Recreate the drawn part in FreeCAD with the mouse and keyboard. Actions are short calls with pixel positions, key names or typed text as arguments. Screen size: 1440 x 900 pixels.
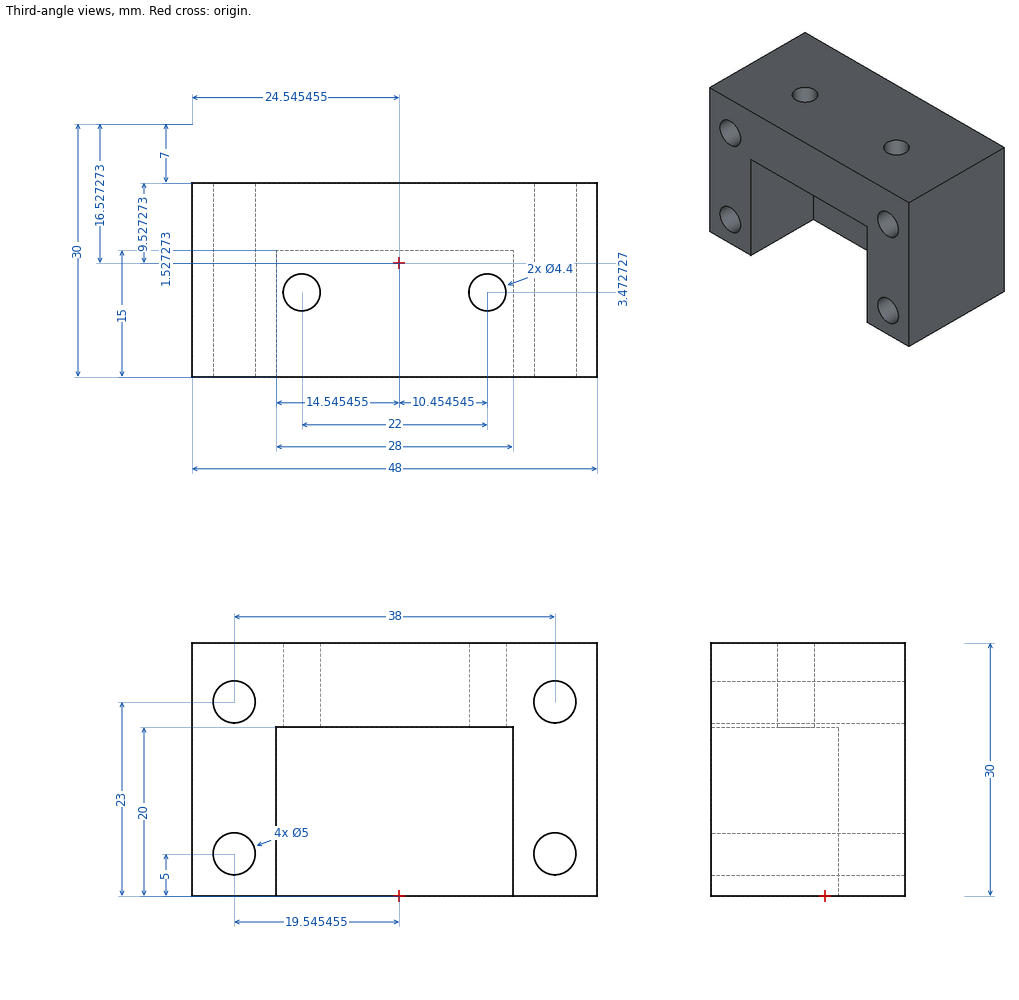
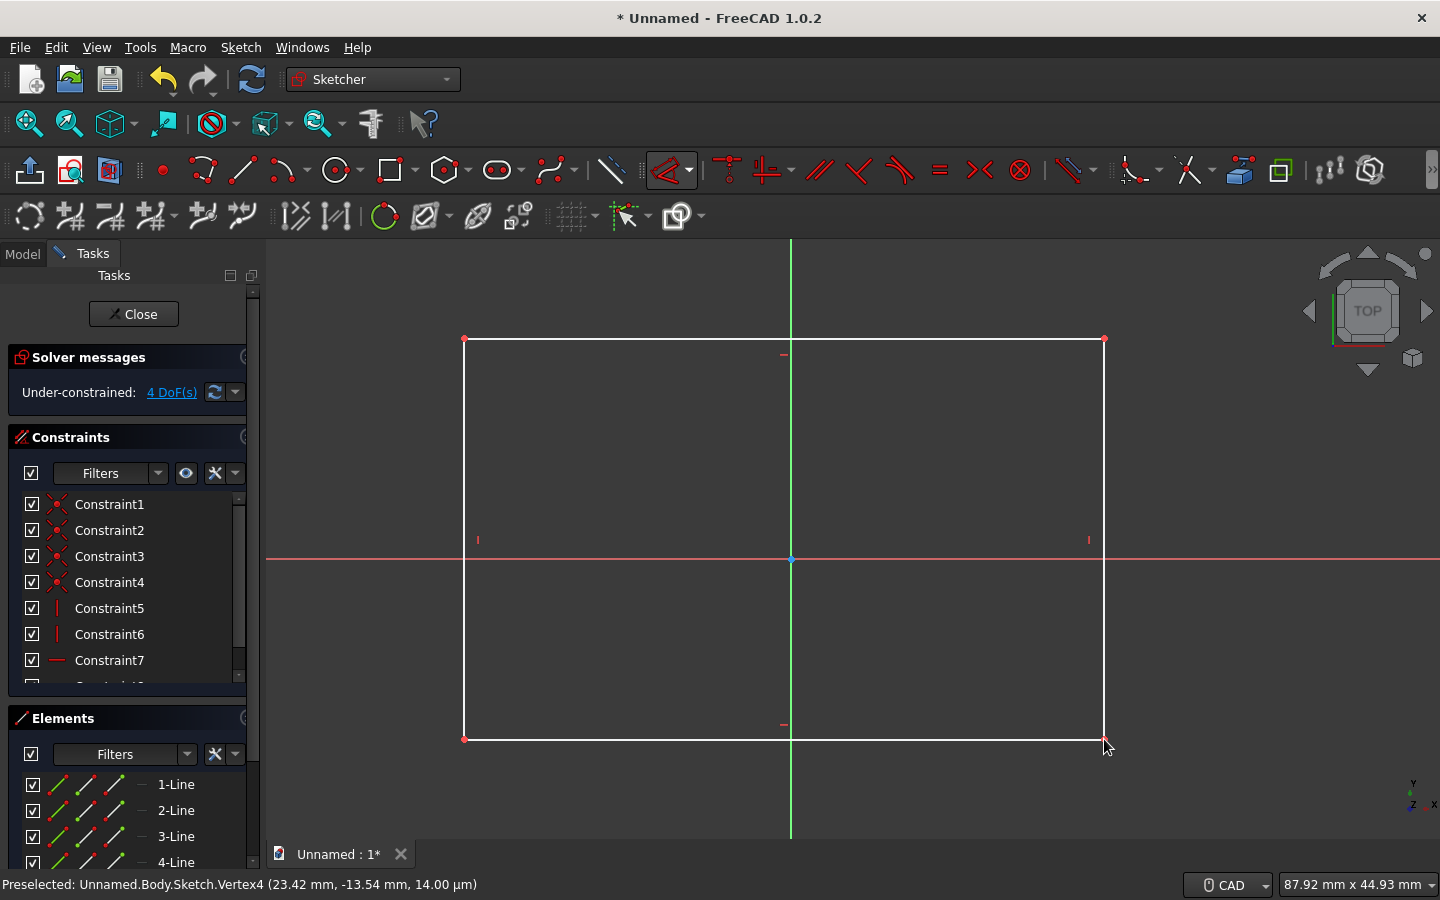
click(666, 170)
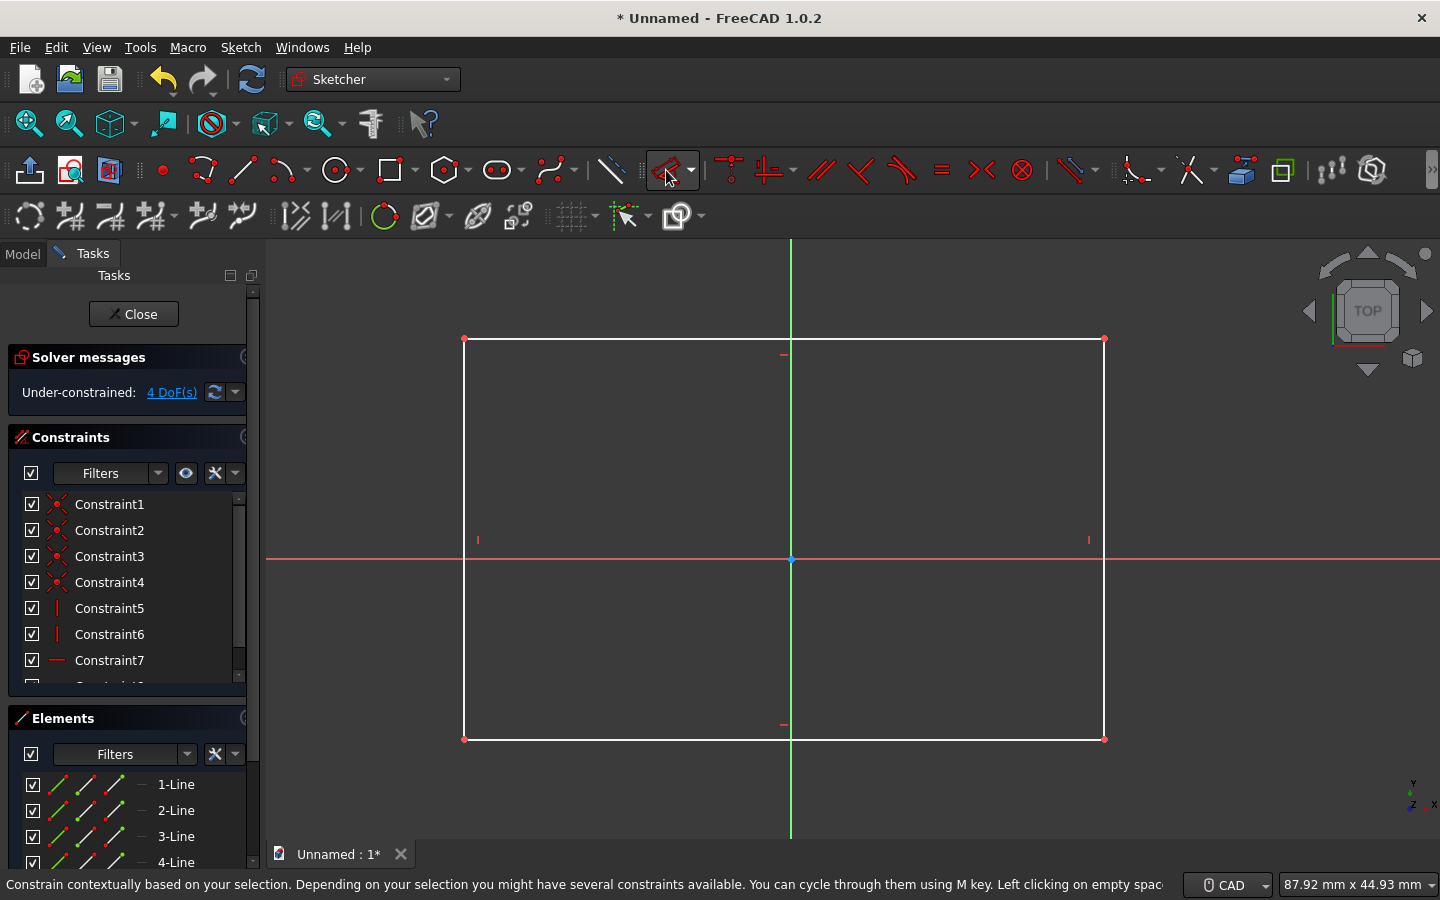
click(464, 459)
click(430, 540)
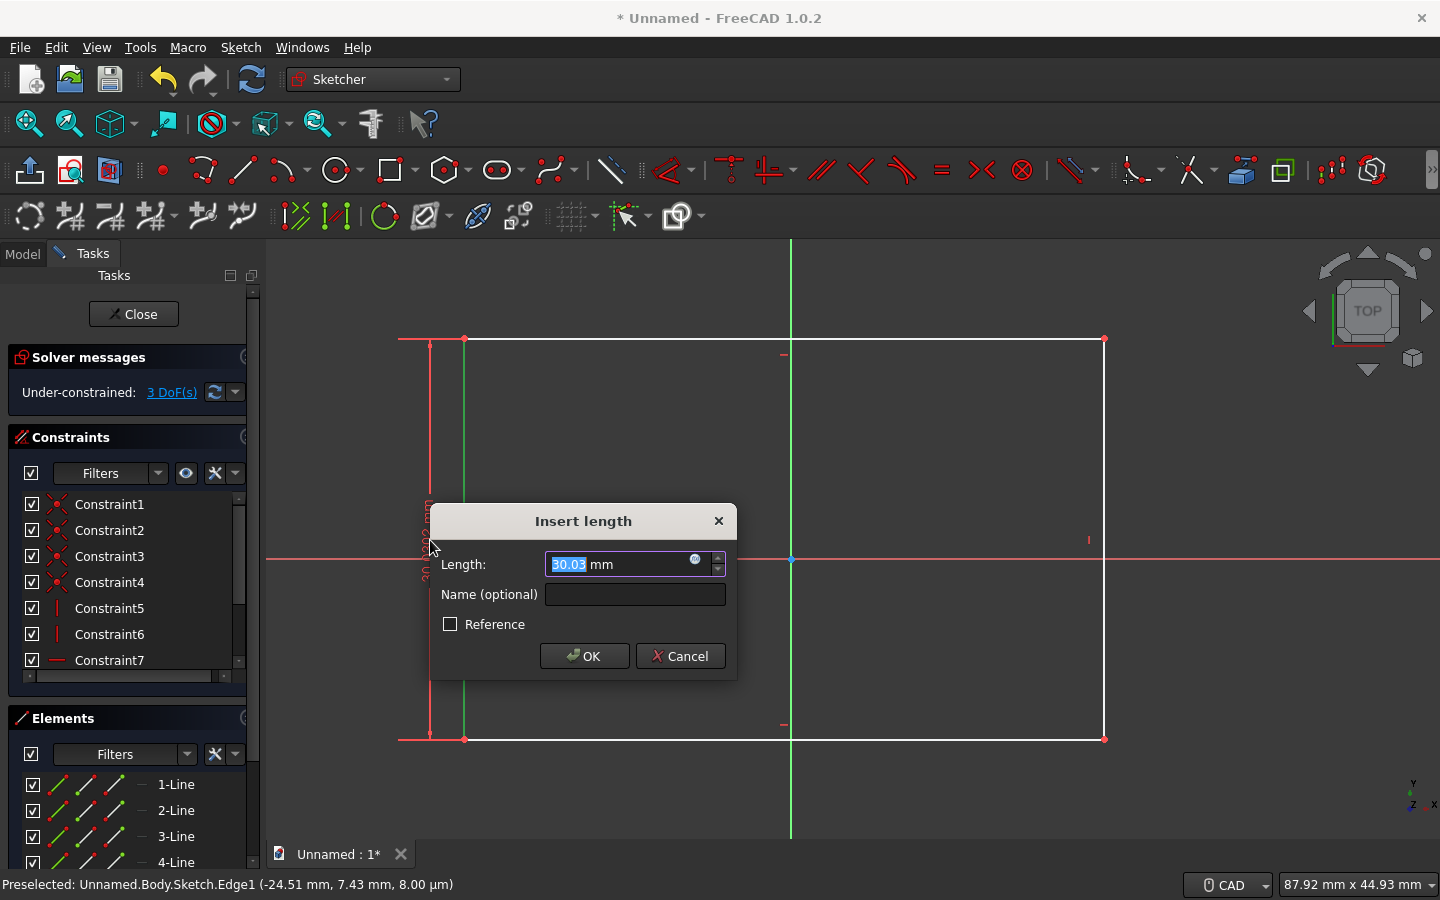
text(30)
key(Return)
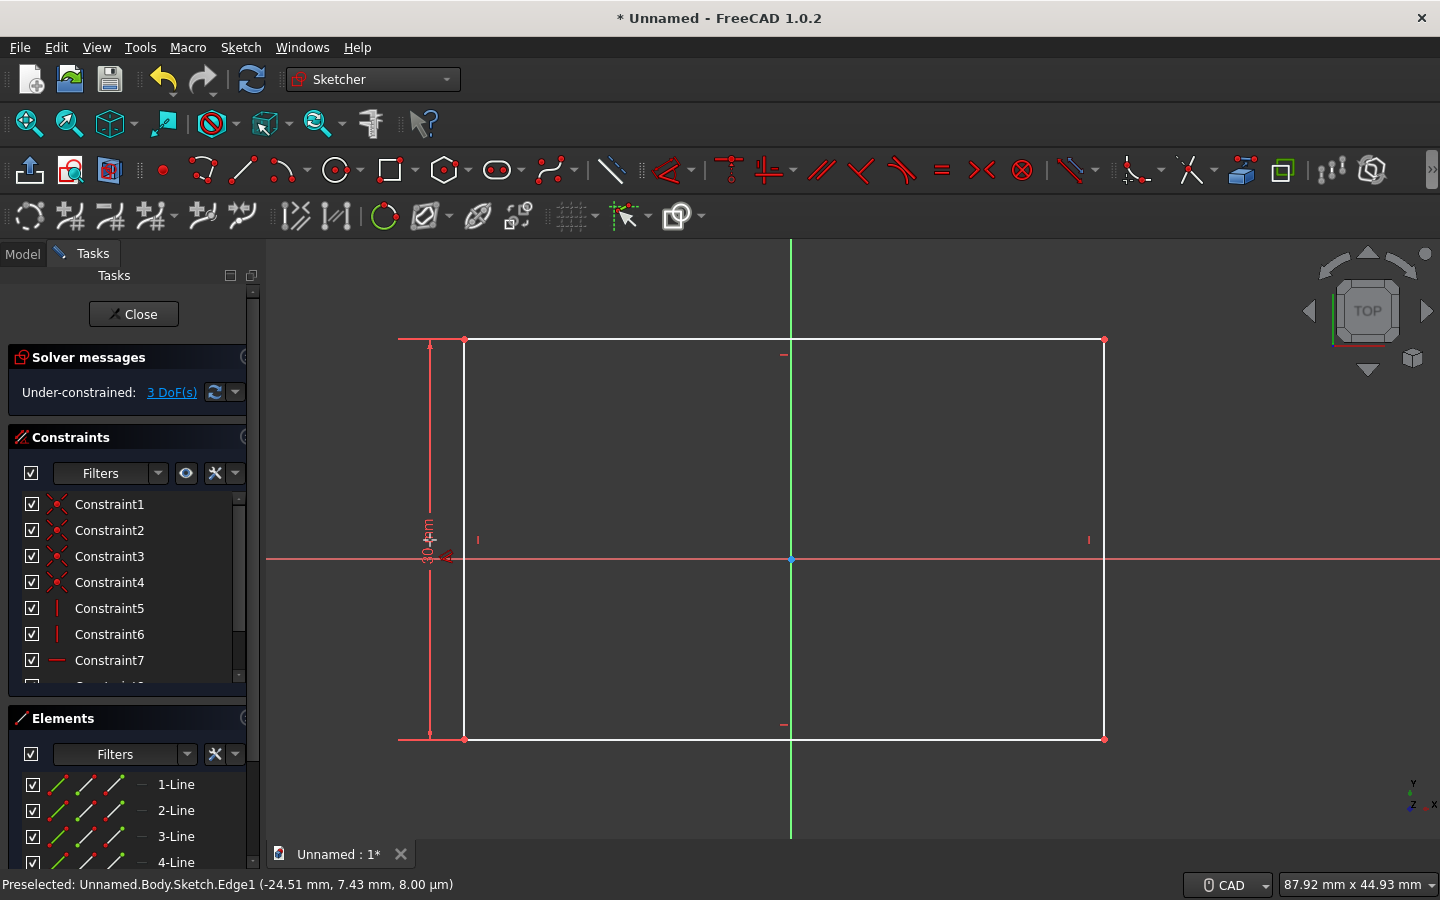
click(656, 740)
click(637, 774)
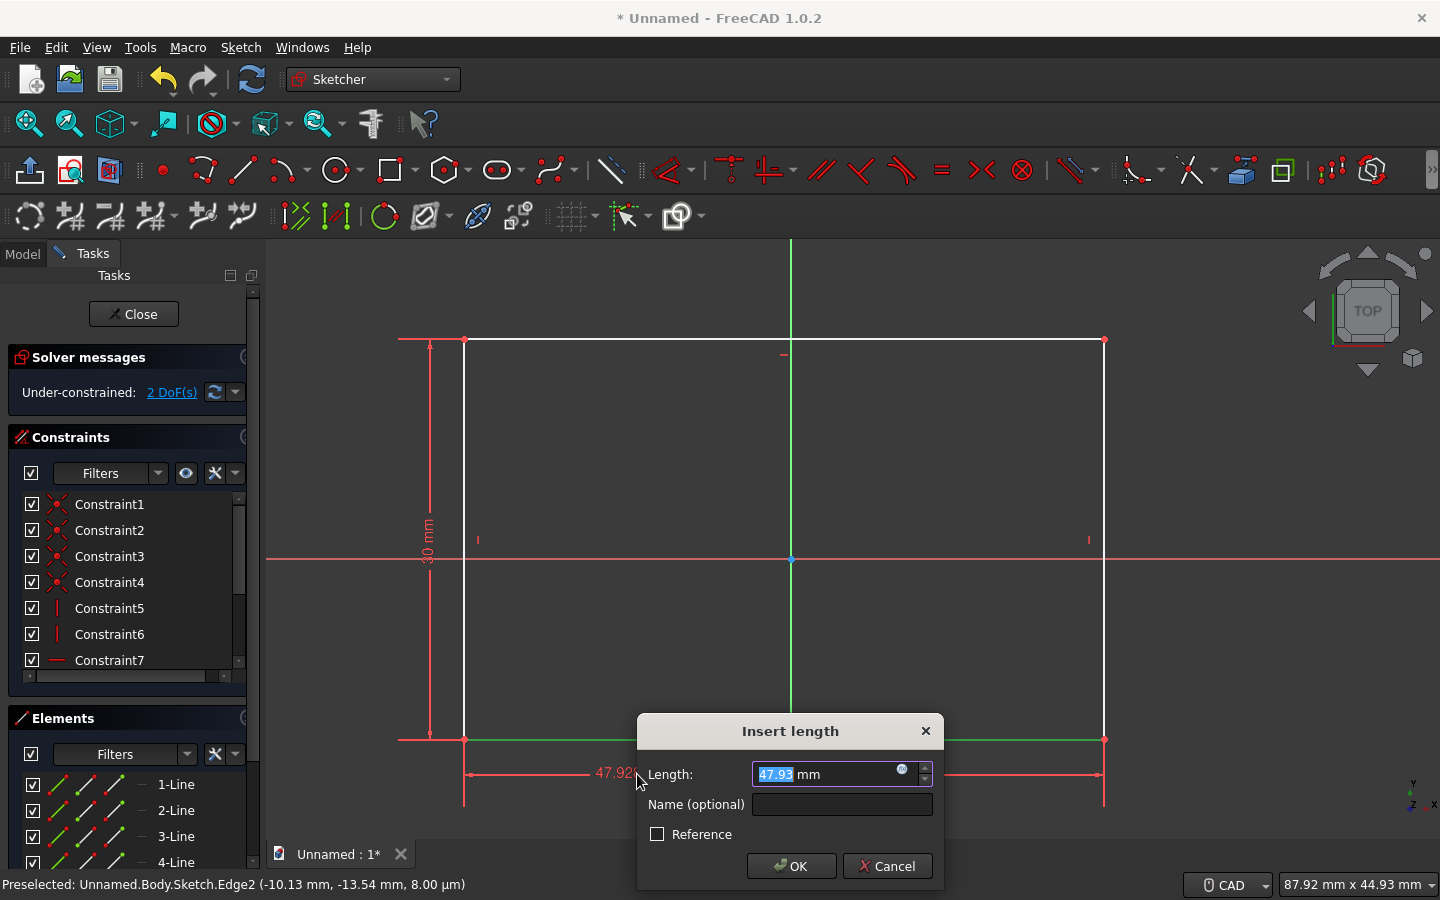
text(48)
key(Return)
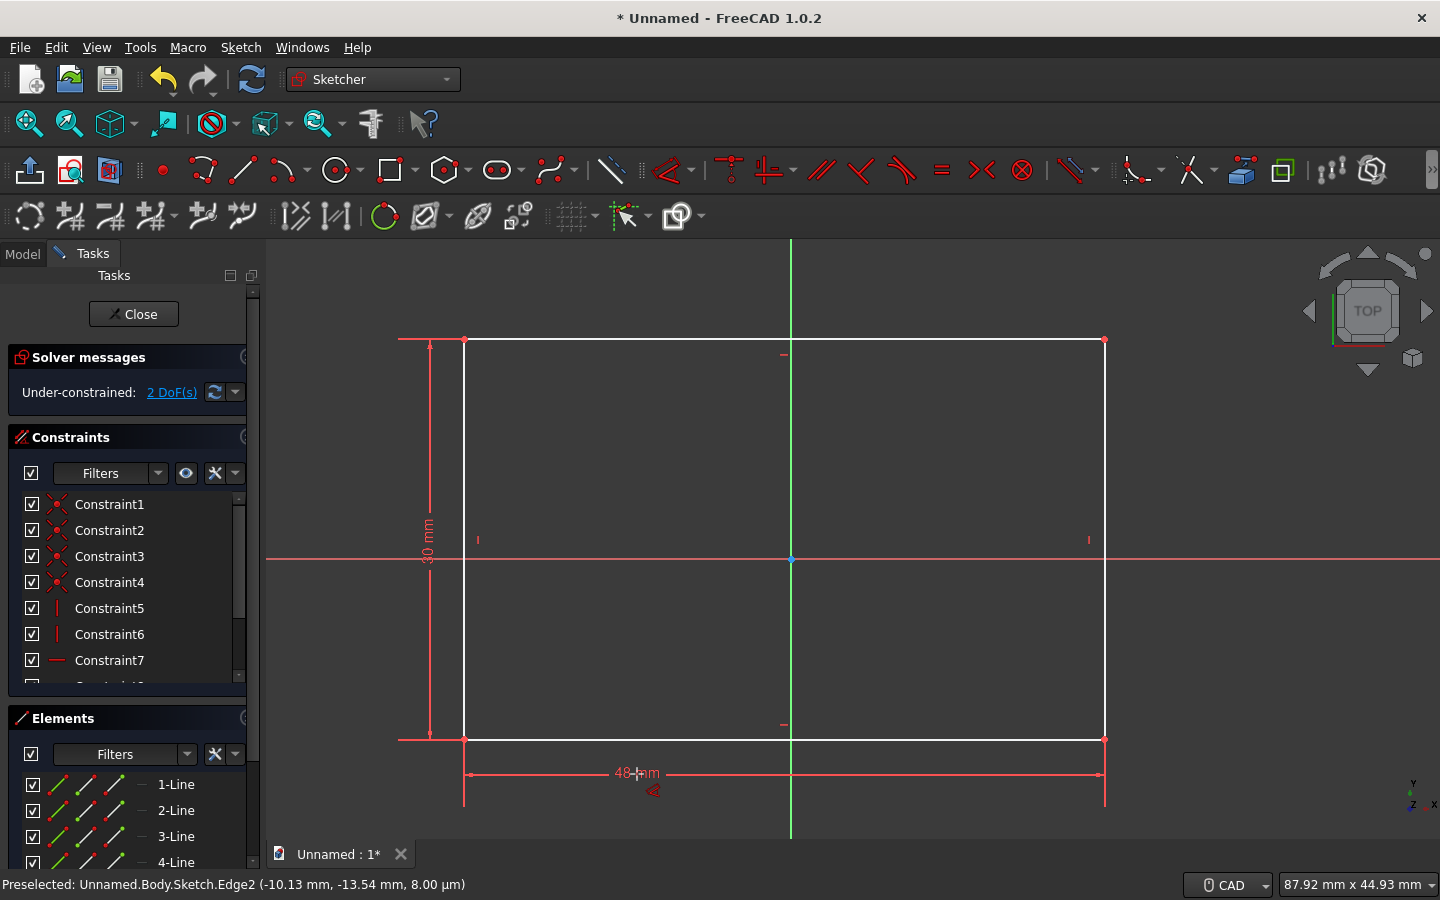
click(464, 339)
click(628, 305)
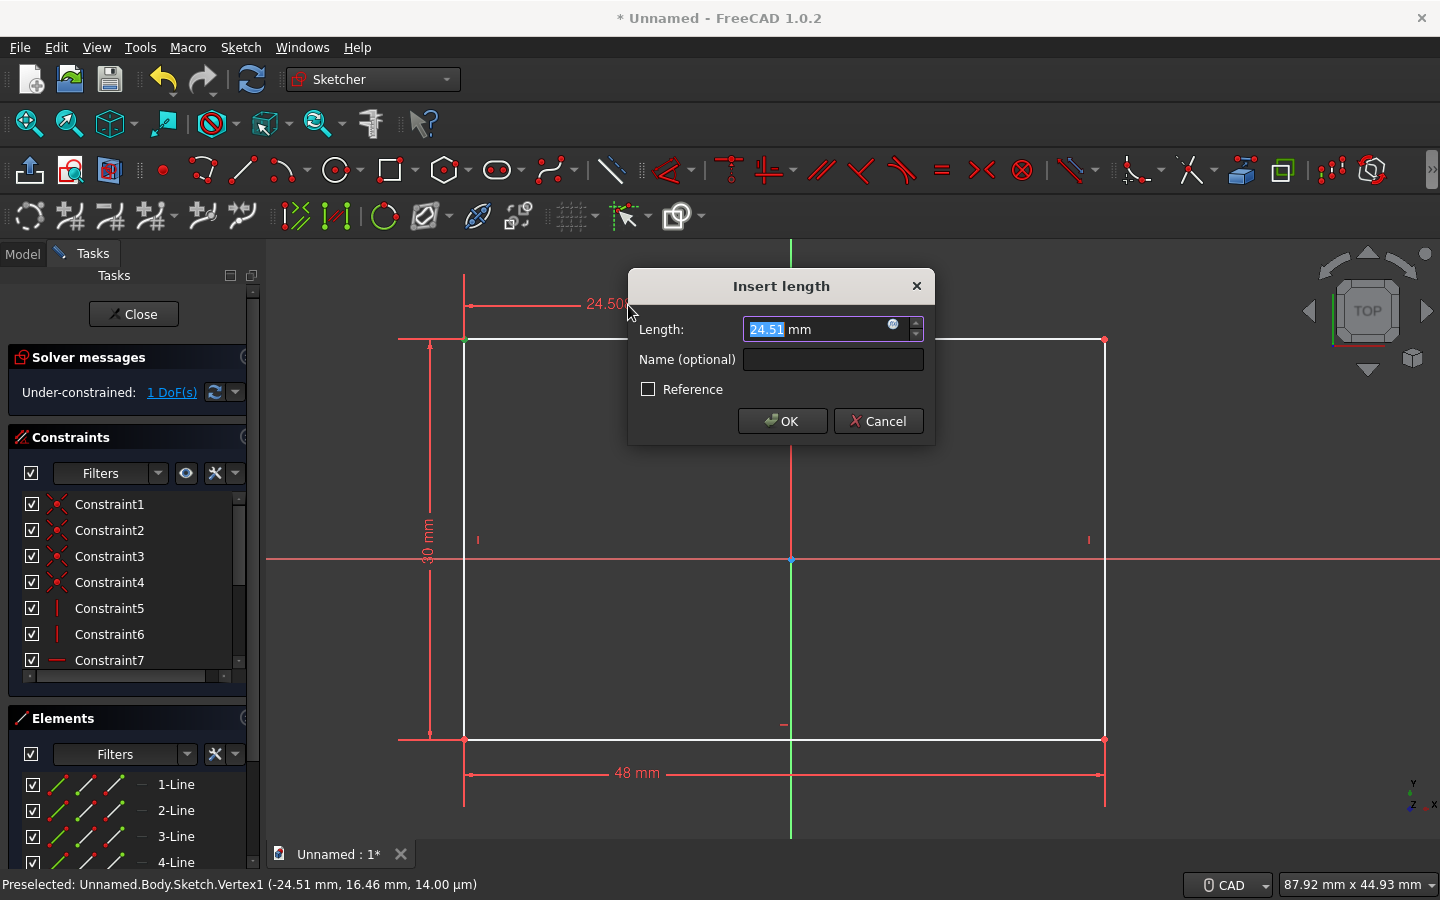
text(24.545455)
key(Return)